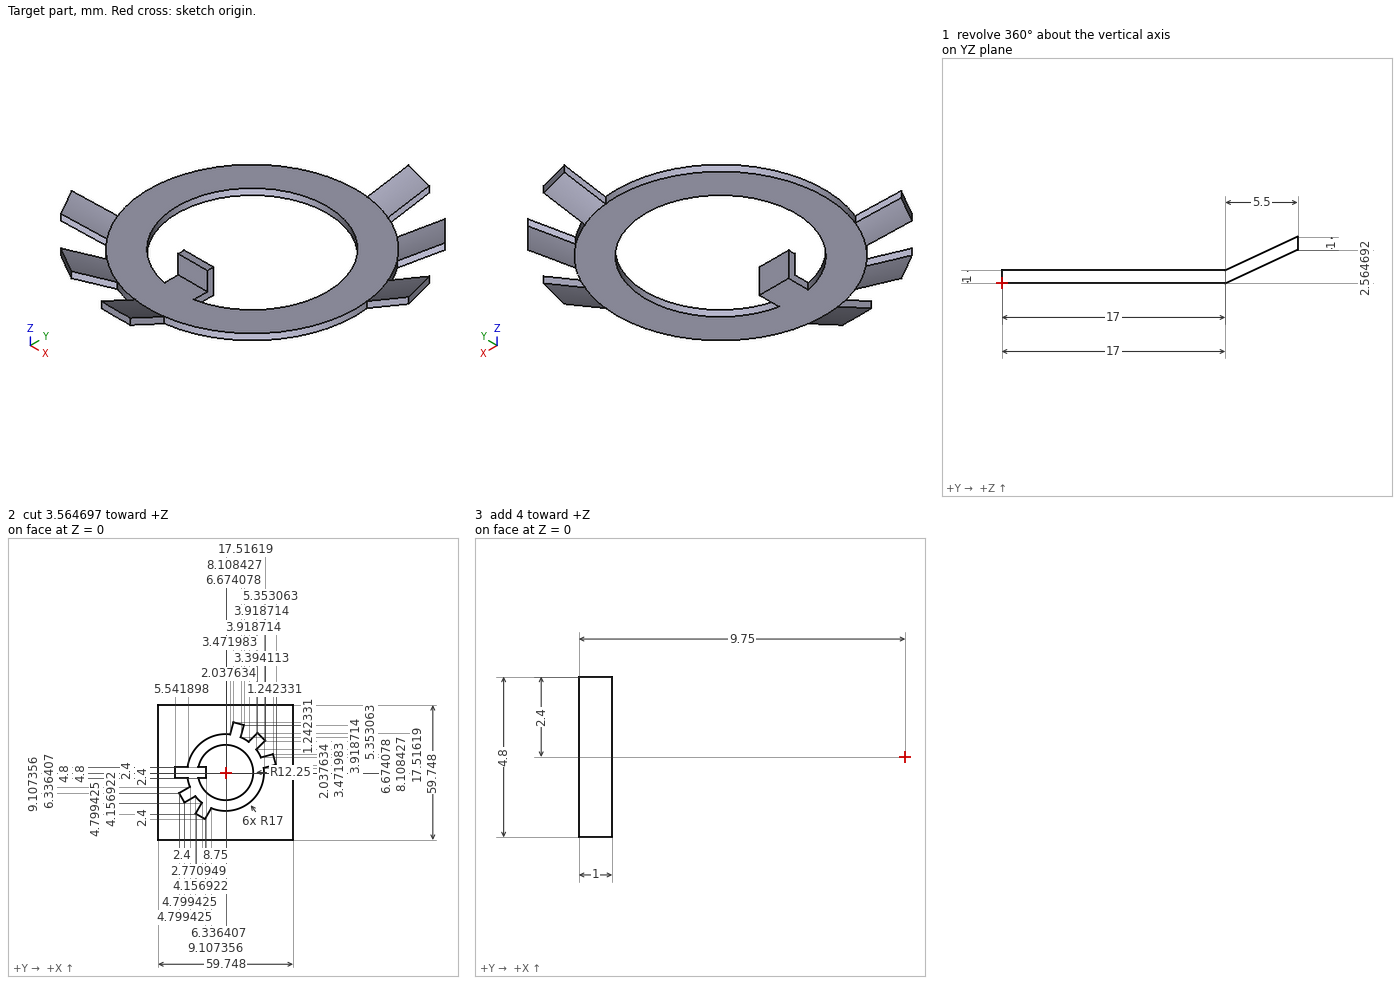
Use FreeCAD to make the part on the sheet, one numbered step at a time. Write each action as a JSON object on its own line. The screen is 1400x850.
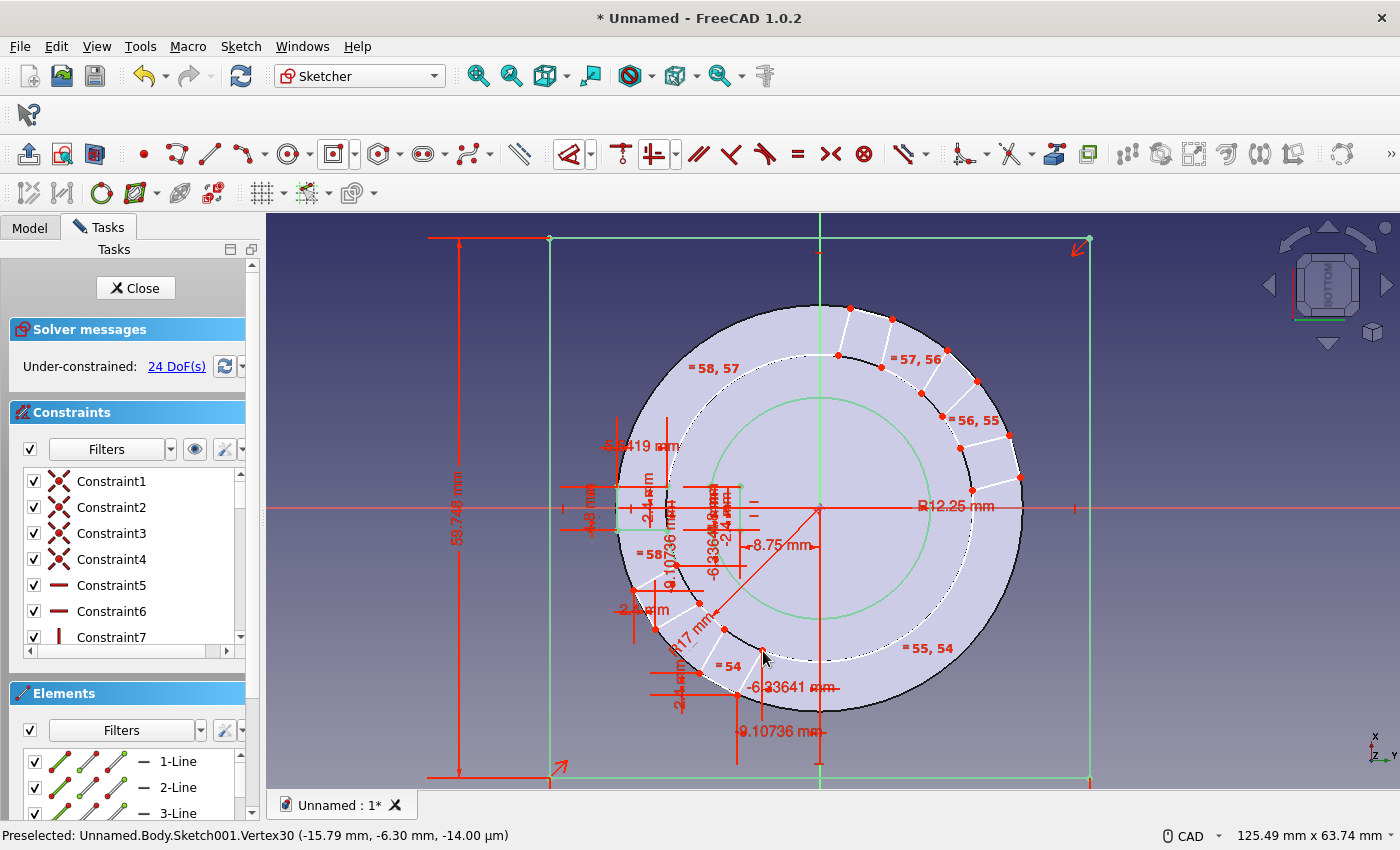
{"action": "scroll", "coordinate": [972, 491], "scroll_direction": "up", "scroll_amount": 4}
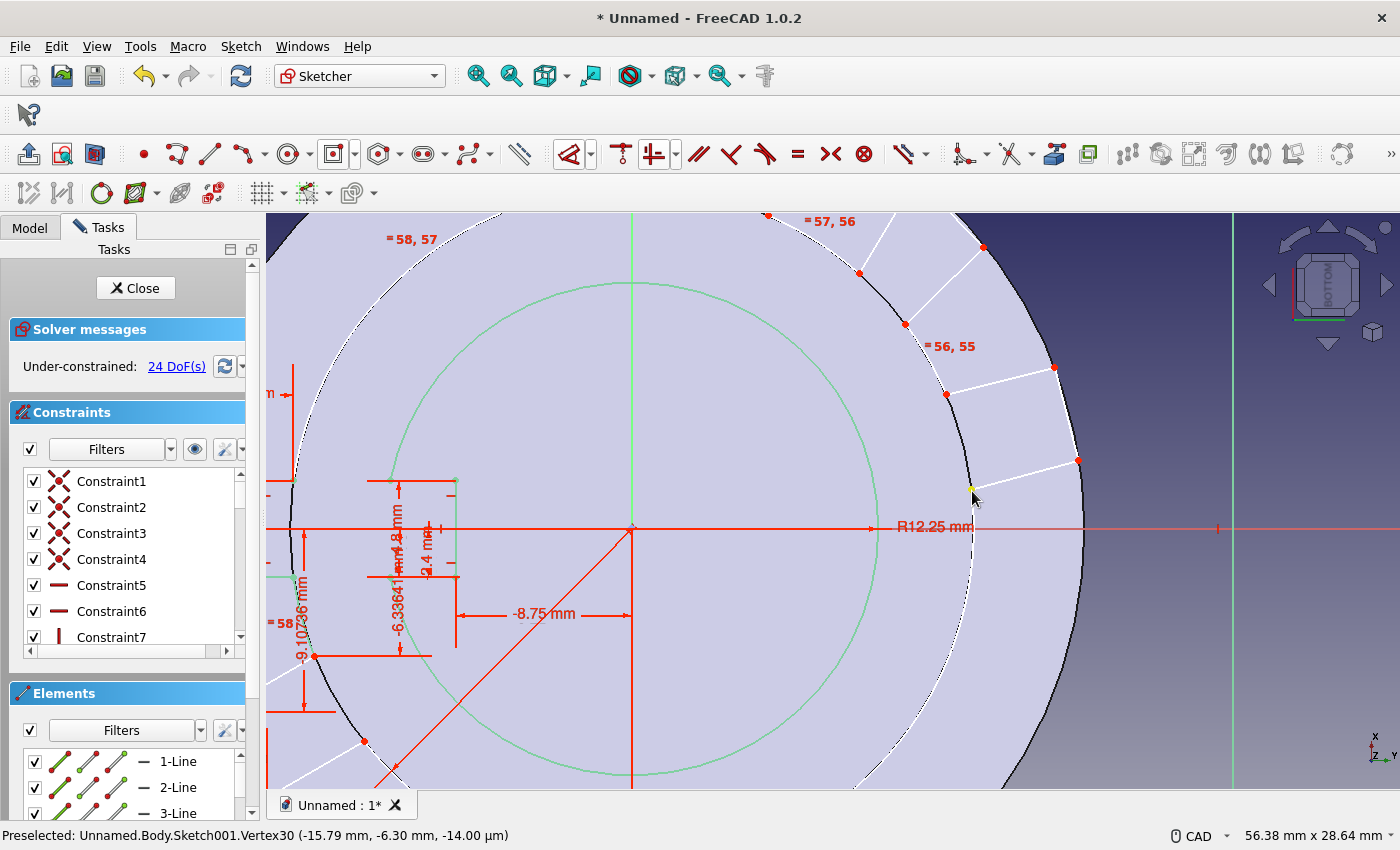
{"action": "left_click", "coordinate": [972, 490]}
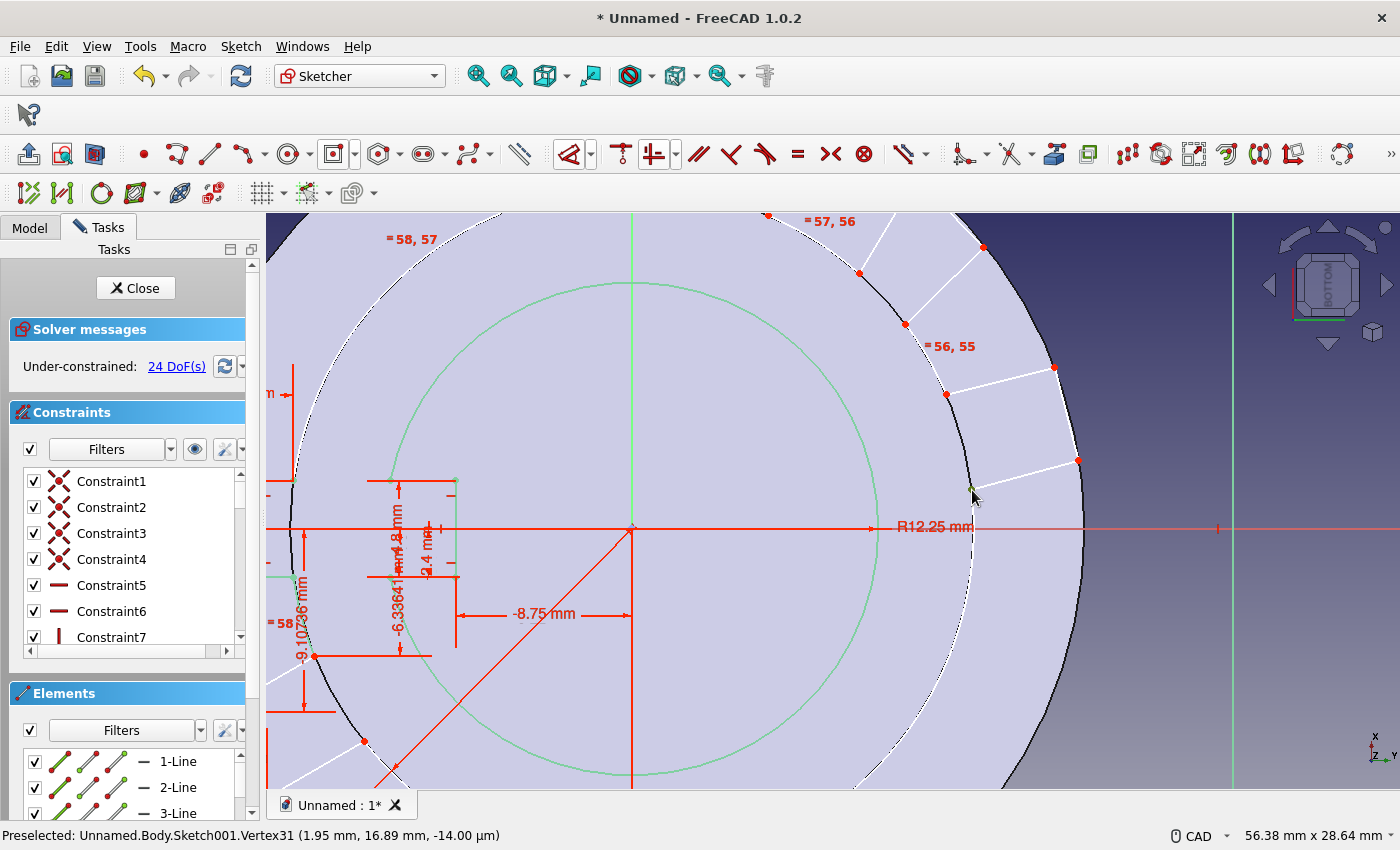
{"action": "left_click", "coordinate": [590, 154]}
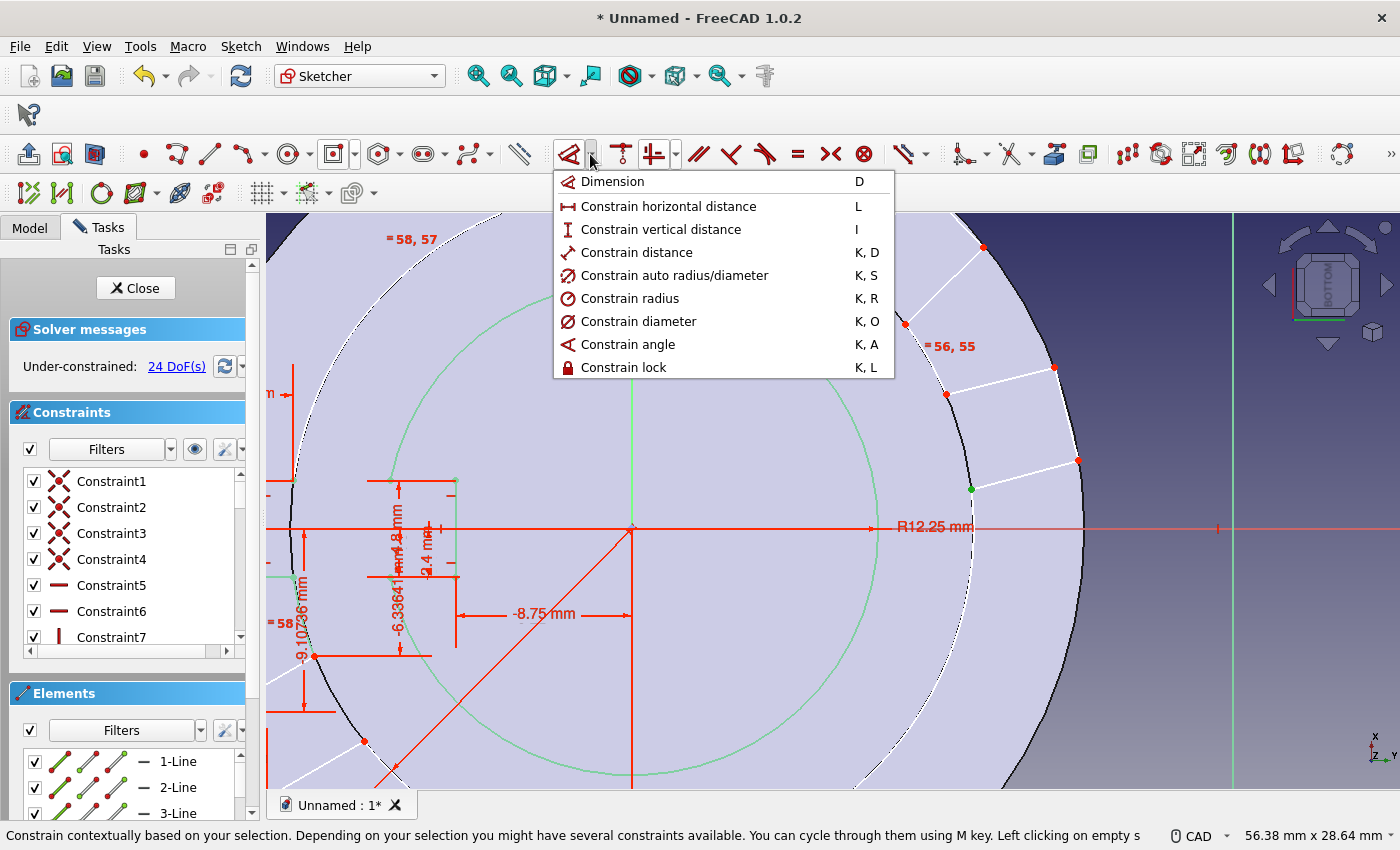
{"action": "left_click", "coordinate": [724, 230]}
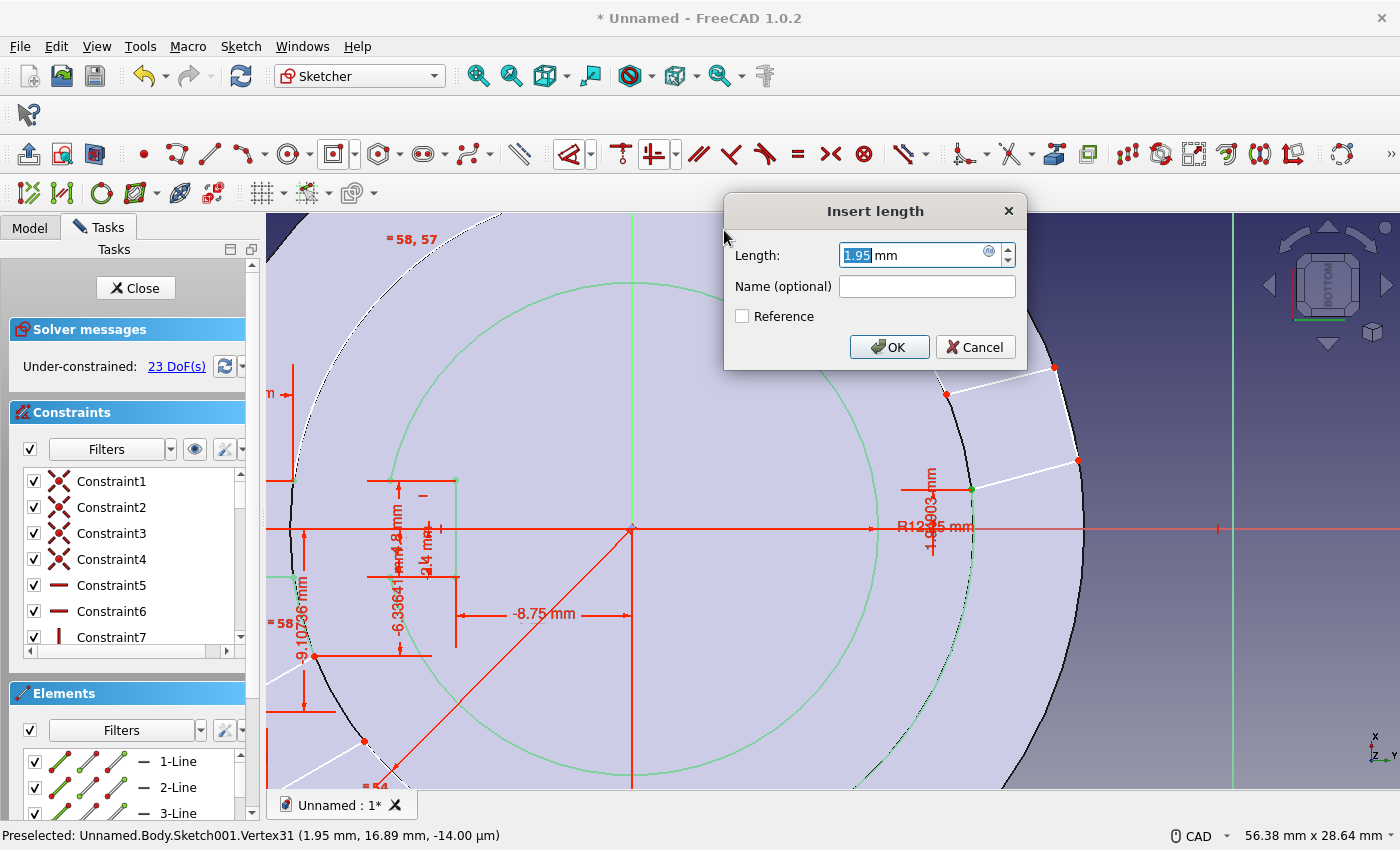
{"action": "type", "text": "2.037634"}
{"action": "key", "text": "Return"}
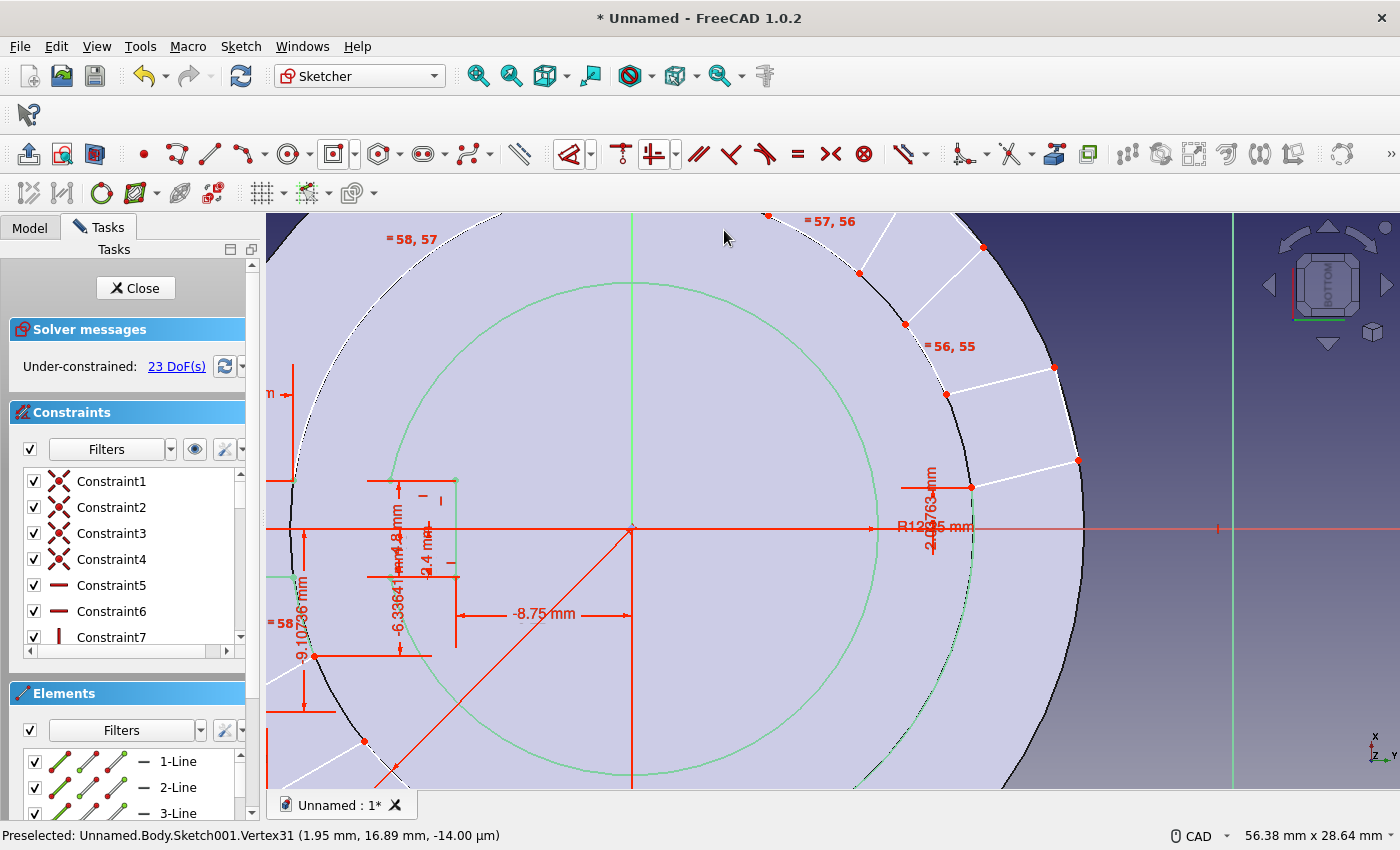
{"action": "left_click", "coordinate": [1079, 461]}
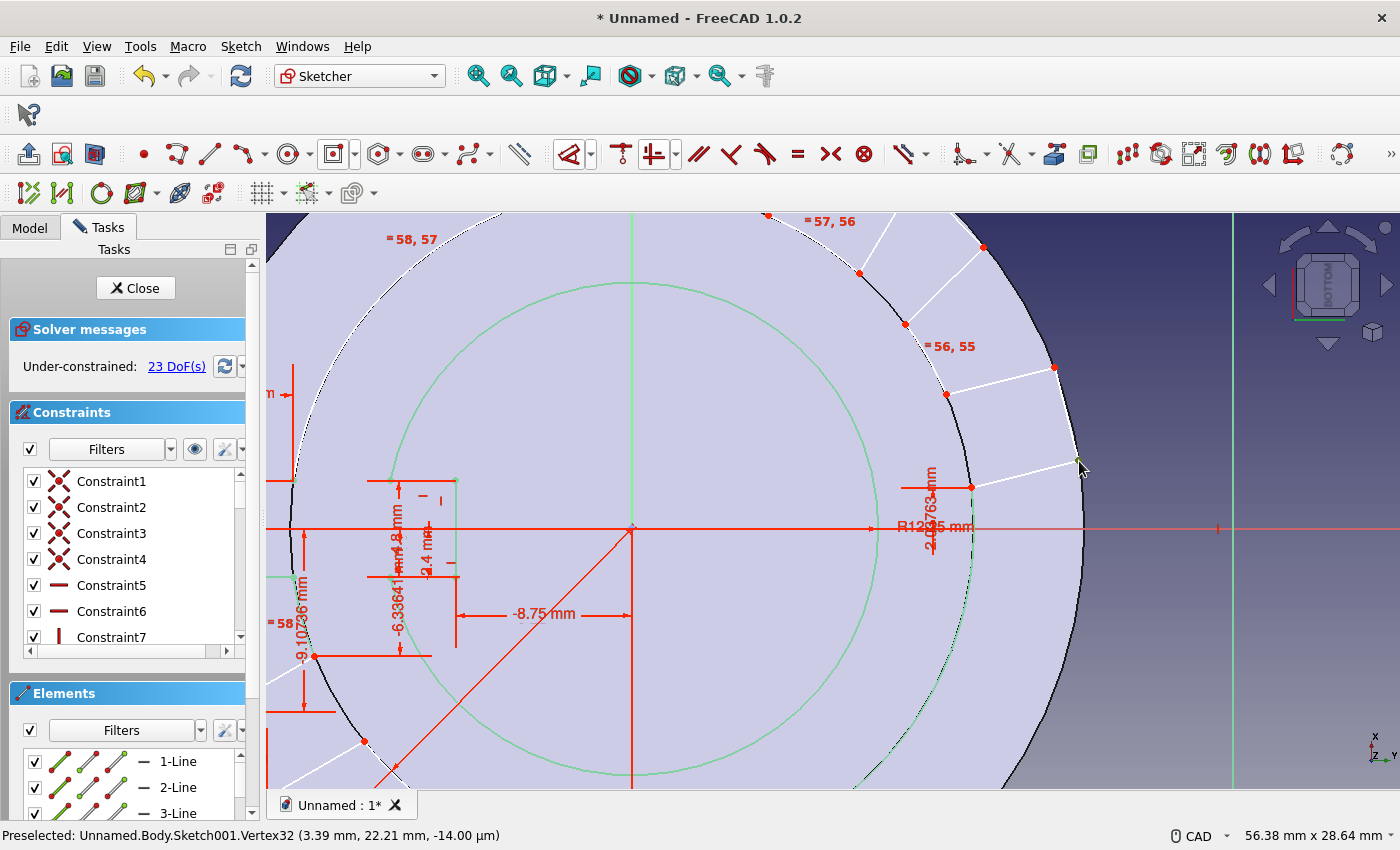
{"action": "key", "text": "i"}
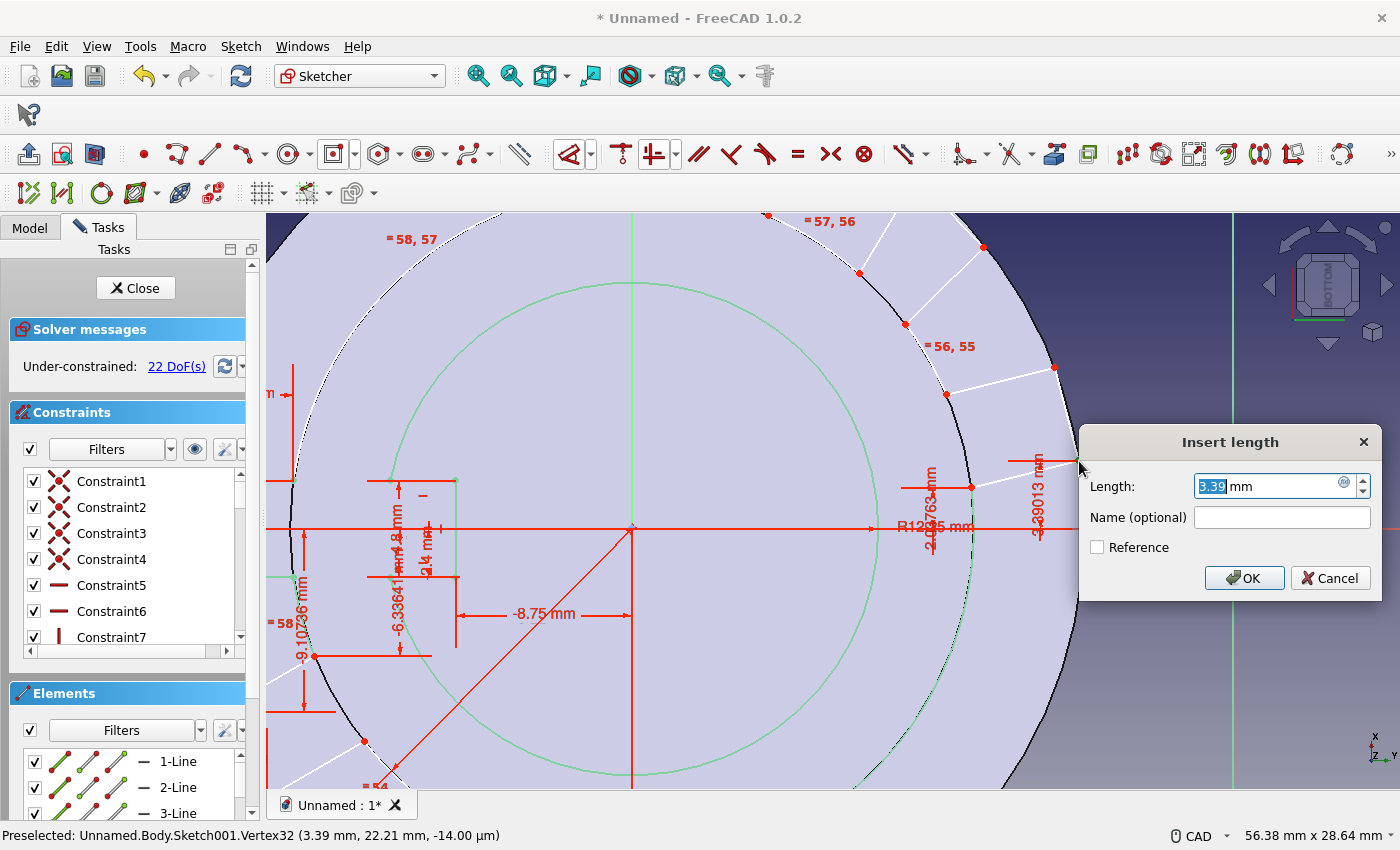
{"action": "type", "text": "3.471983"}
{"action": "key", "text": "Return"}